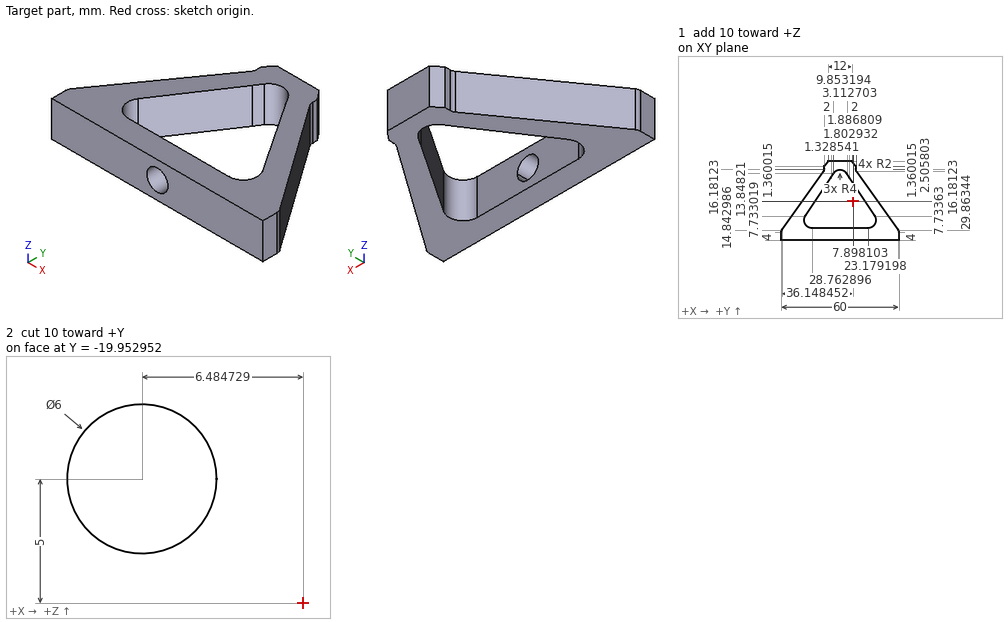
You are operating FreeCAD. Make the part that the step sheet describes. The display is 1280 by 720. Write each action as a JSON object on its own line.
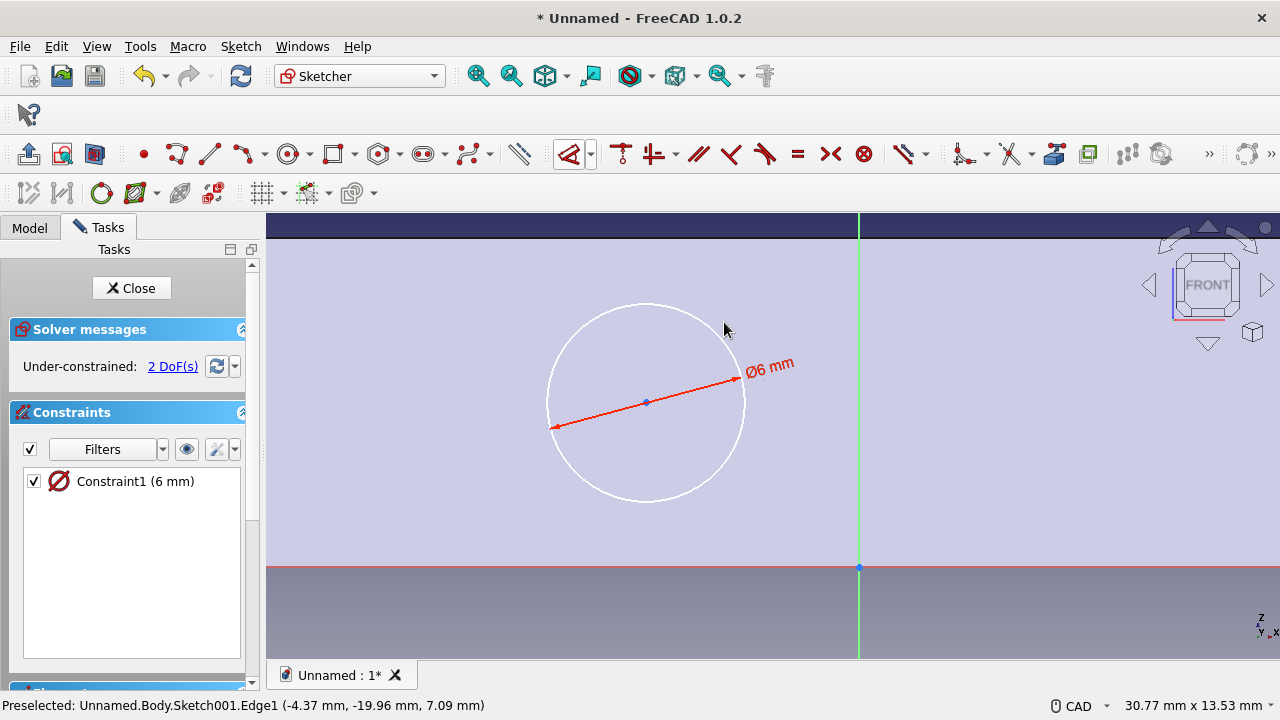
{"action": "left_click", "coordinate": [646, 403]}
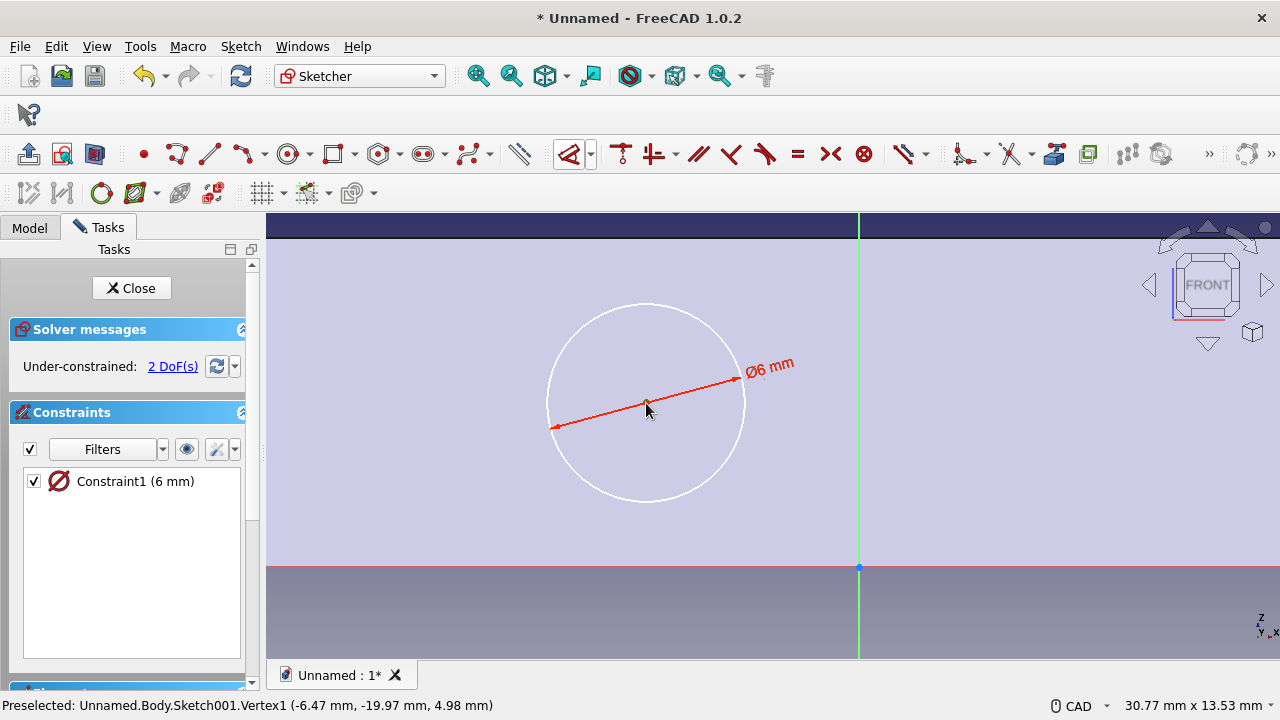
{"action": "key", "text": "i"}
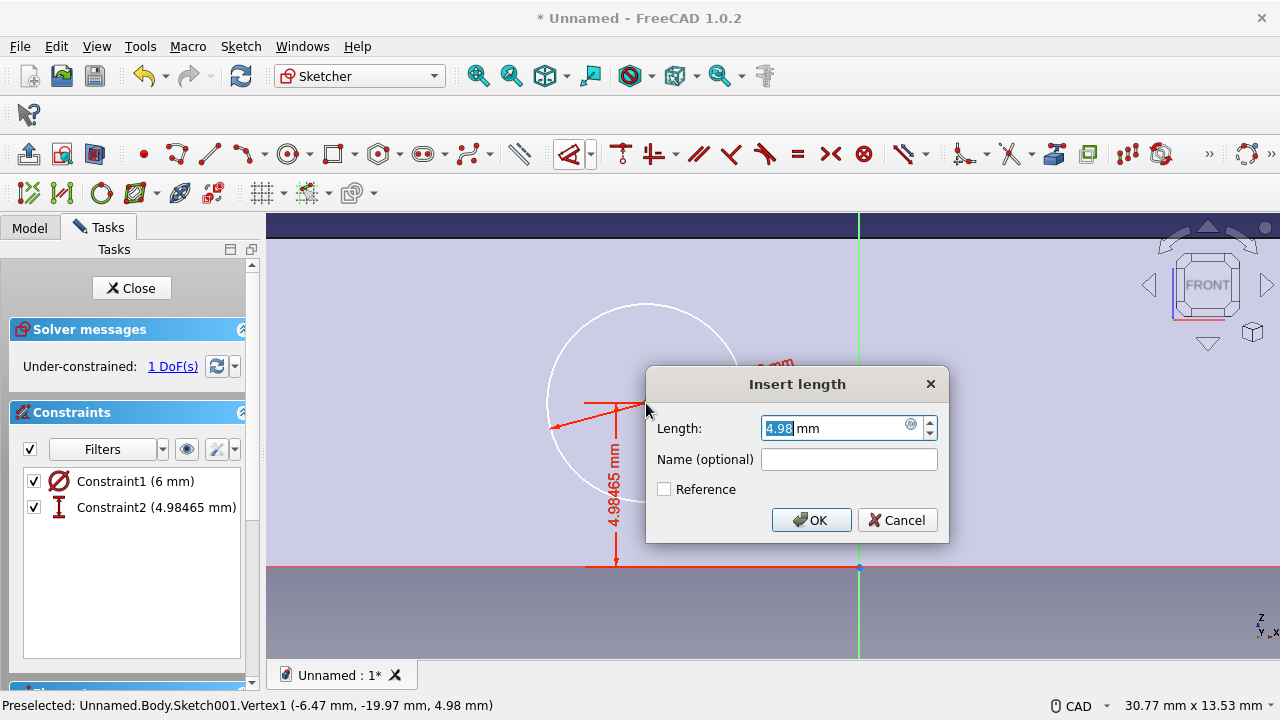
{"action": "type", "text": "5"}
{"action": "key", "text": "Return"}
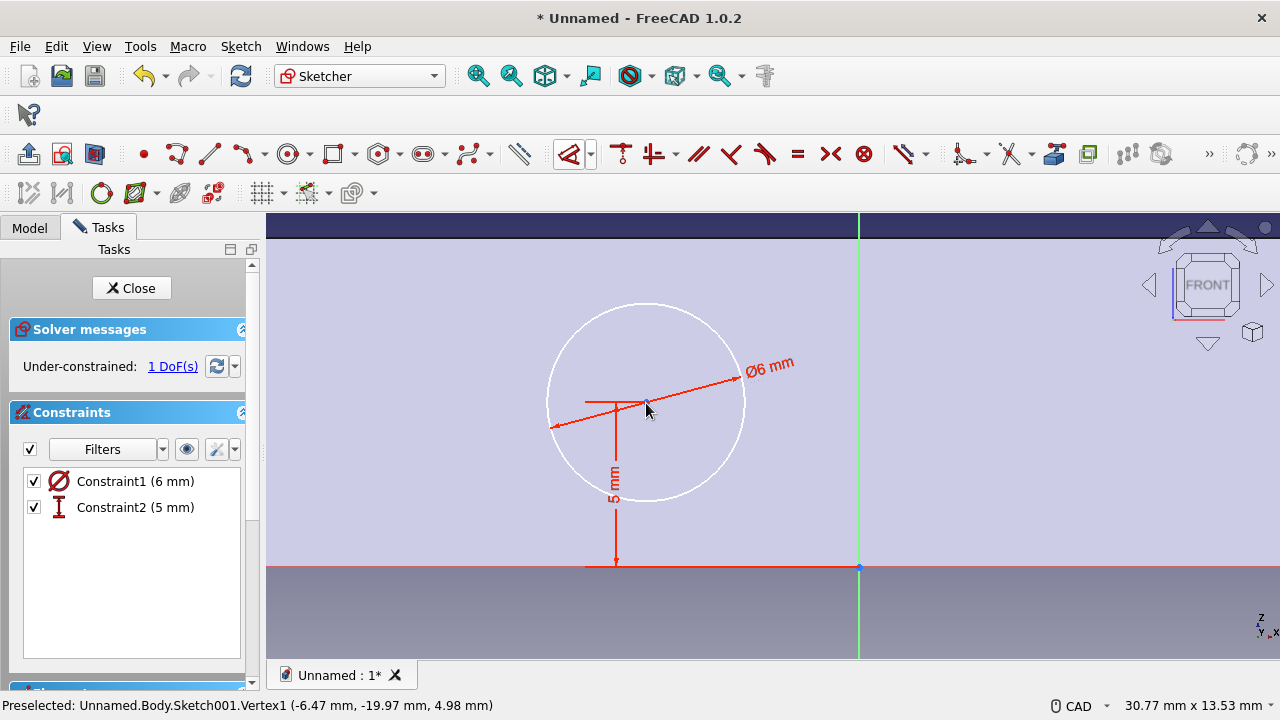
{"action": "left_click", "coordinate": [646, 402]}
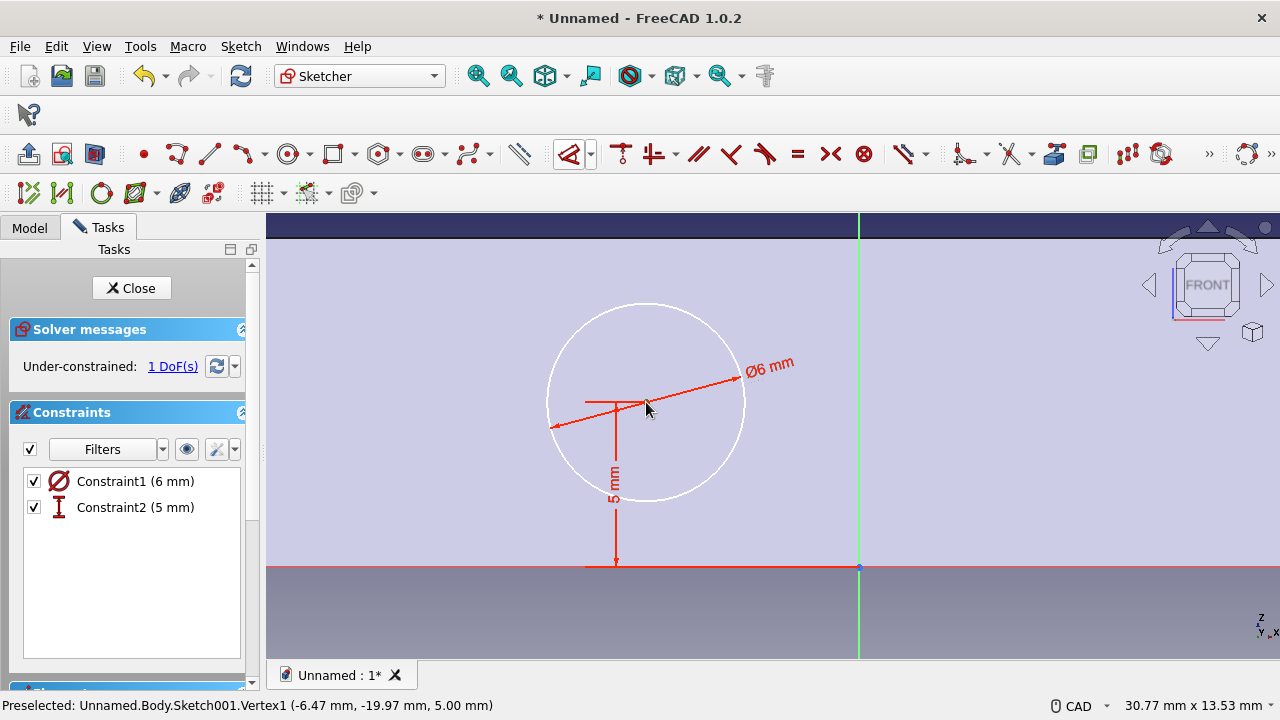
{"action": "left_click", "coordinate": [590, 154]}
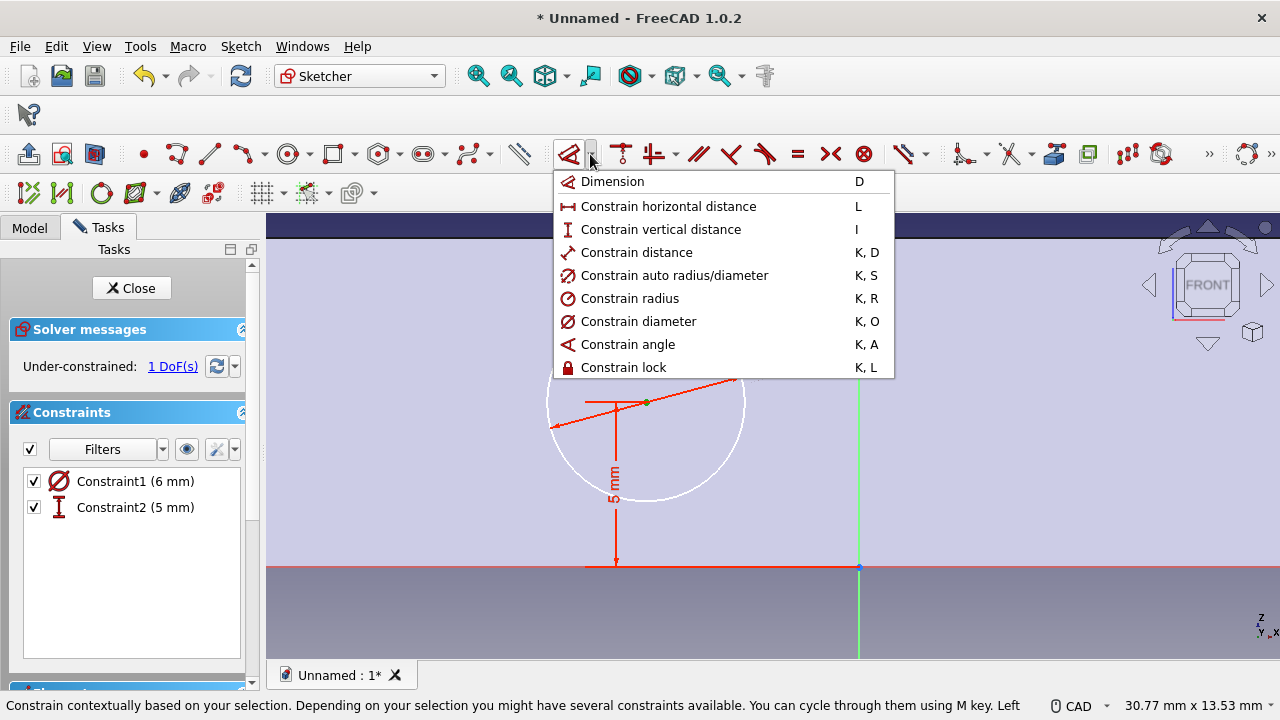
{"action": "left_click", "coordinate": [724, 206]}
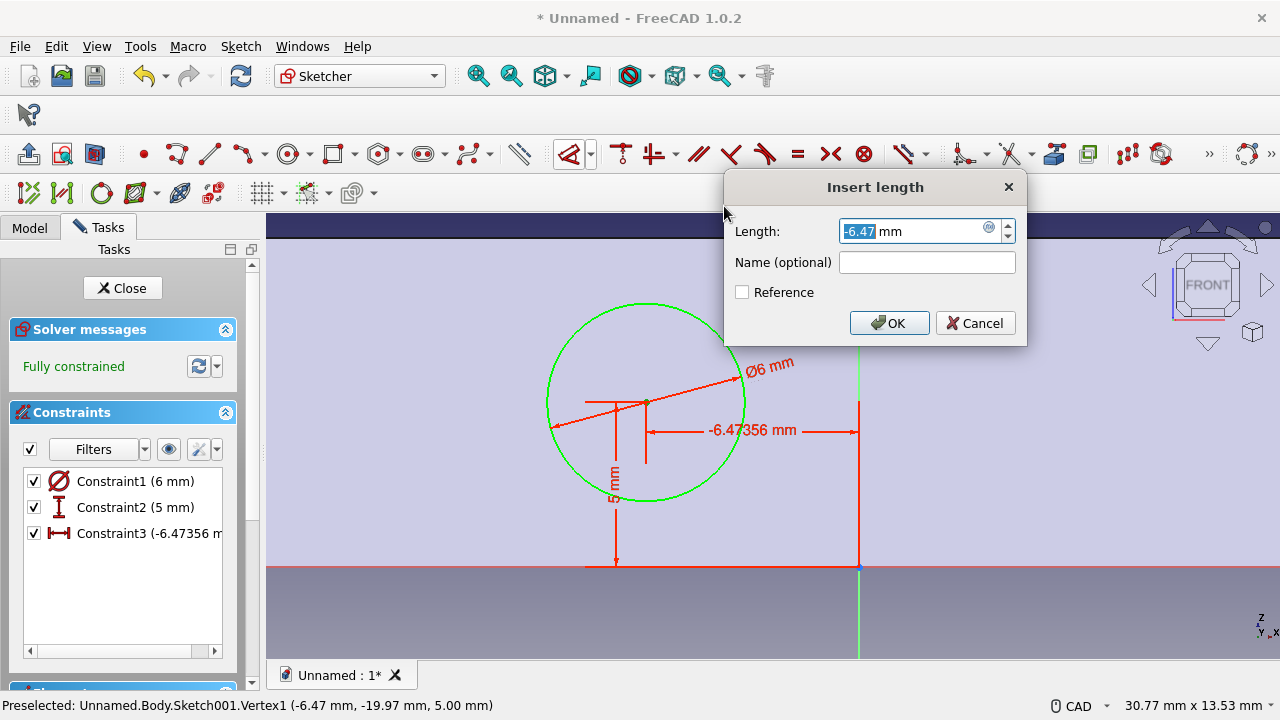
{"action": "type", "text": "-6.484729"}
{"action": "key", "text": "Return"}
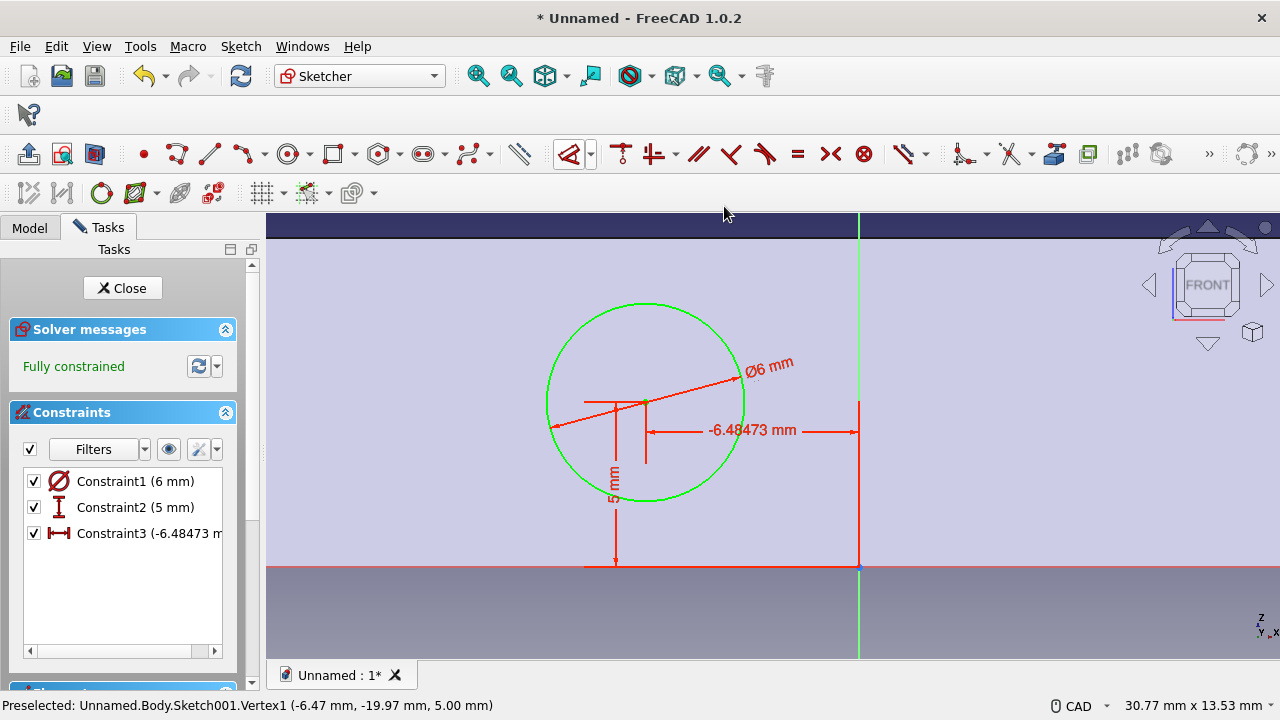
{"action": "left_click", "coordinate": [123, 288]}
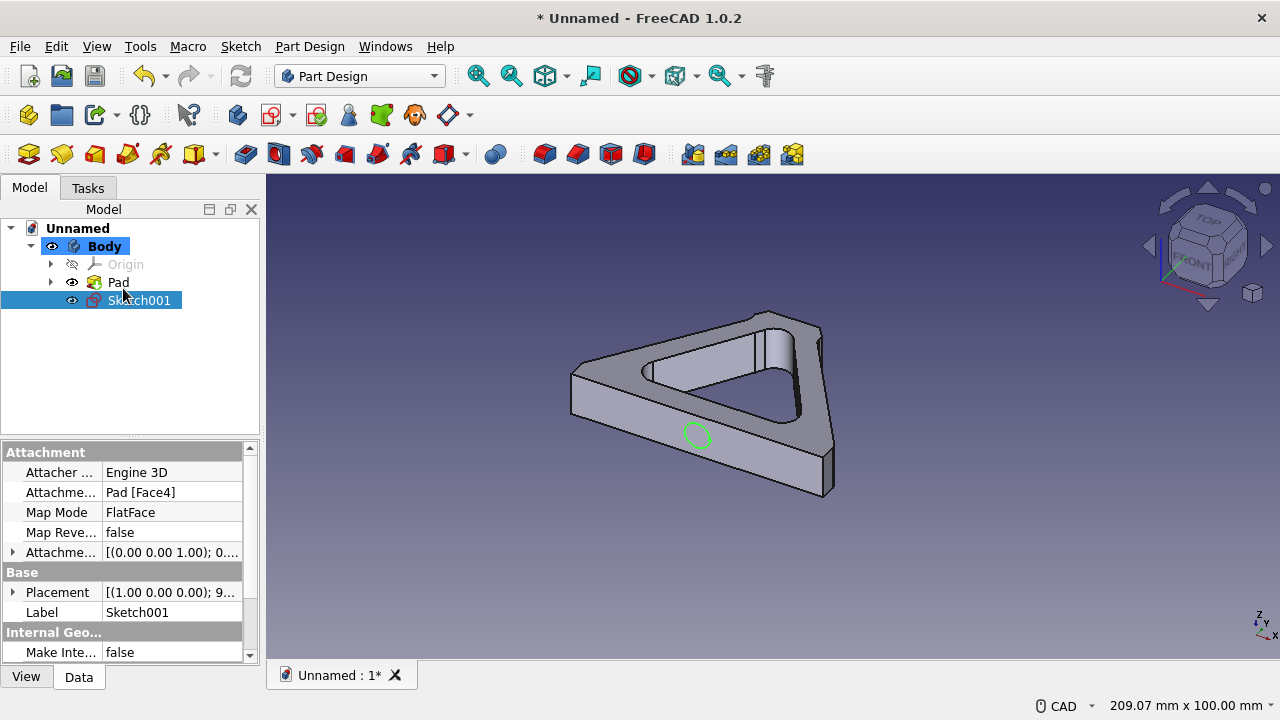
{"action": "left_click", "coordinate": [246, 154]}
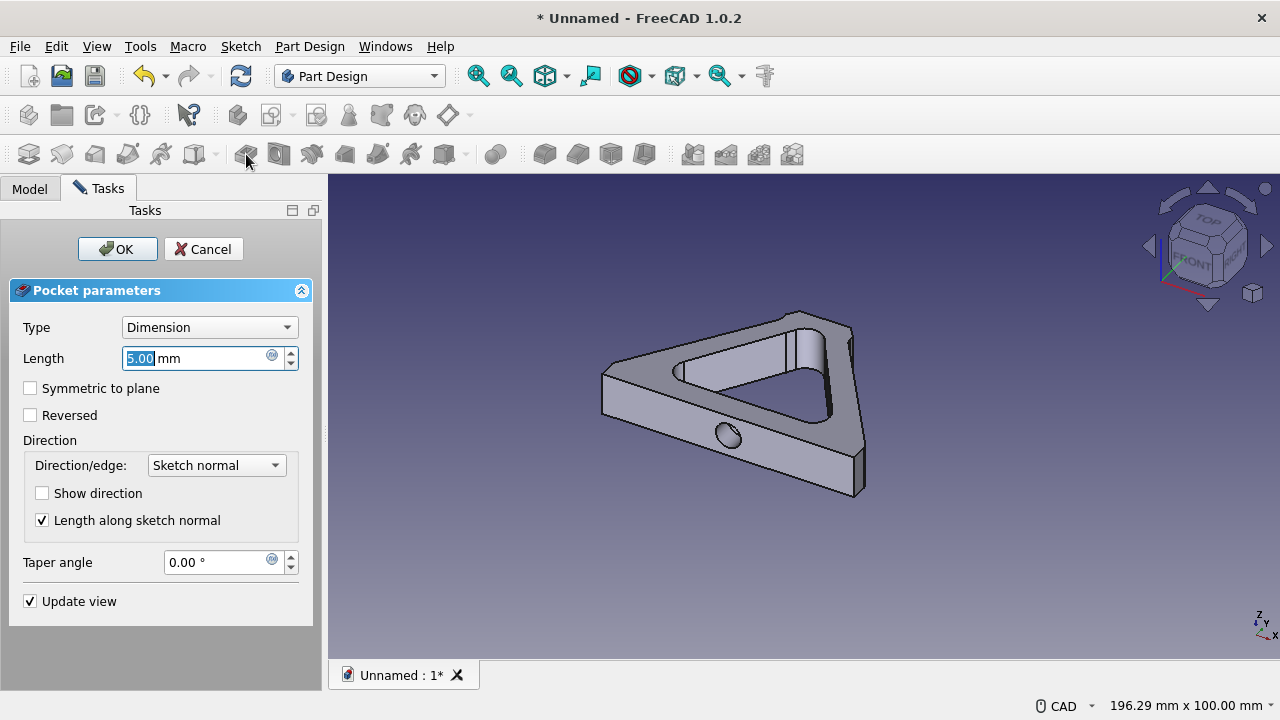
{"action": "type", "text": "10"}
{"action": "key", "text": "Tab"}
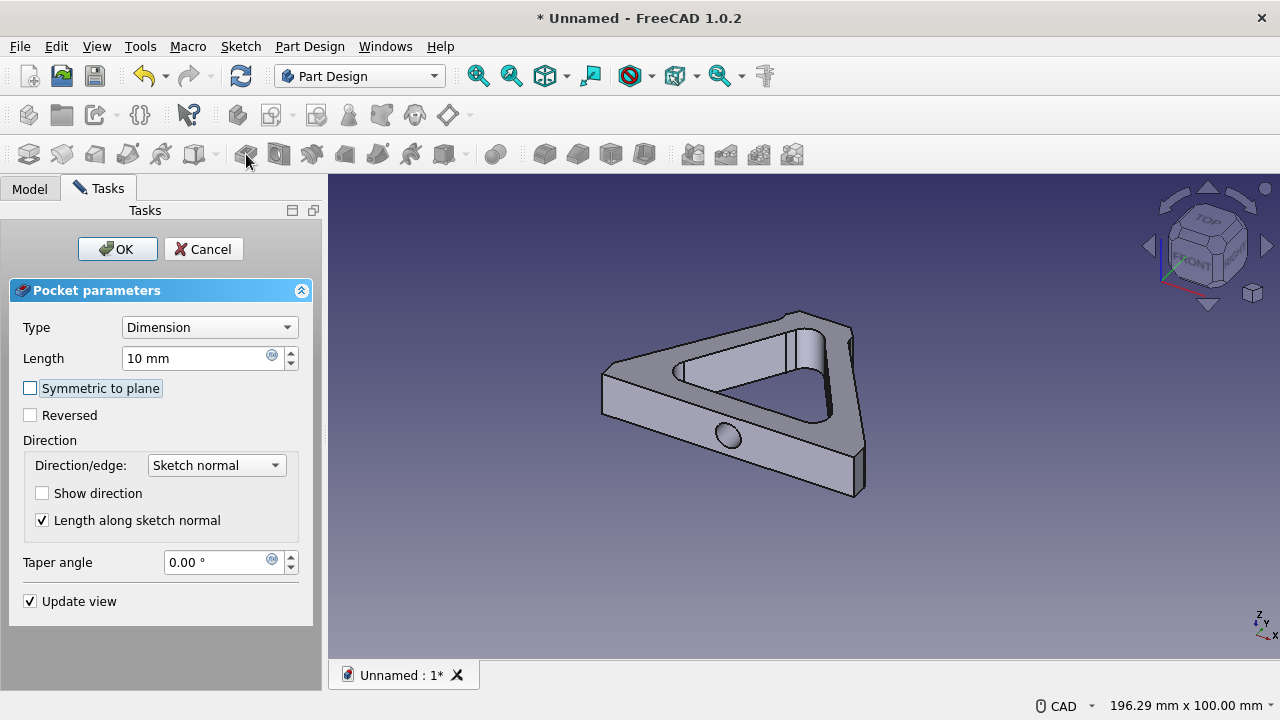
{"action": "left_click", "coordinate": [118, 249]}